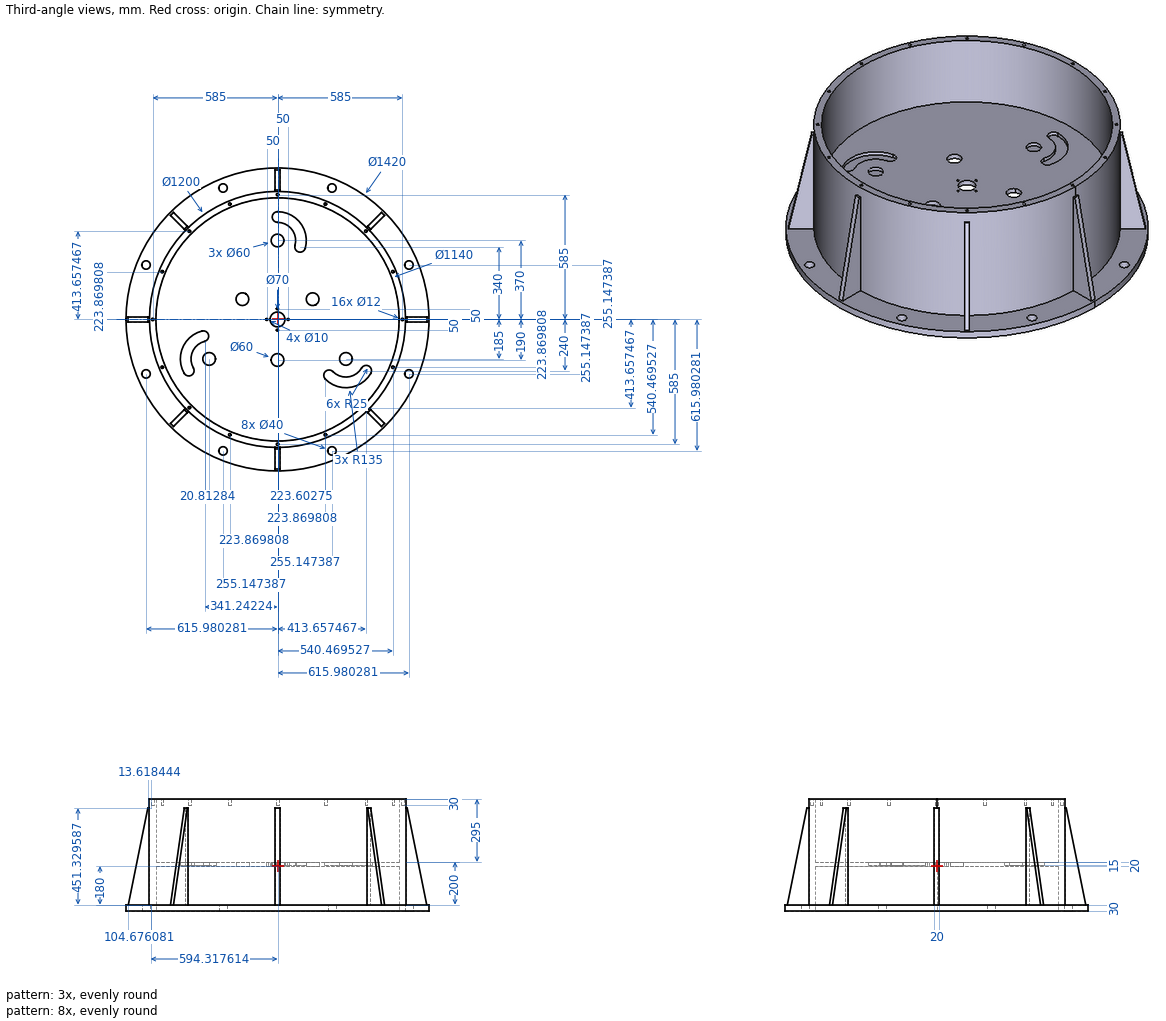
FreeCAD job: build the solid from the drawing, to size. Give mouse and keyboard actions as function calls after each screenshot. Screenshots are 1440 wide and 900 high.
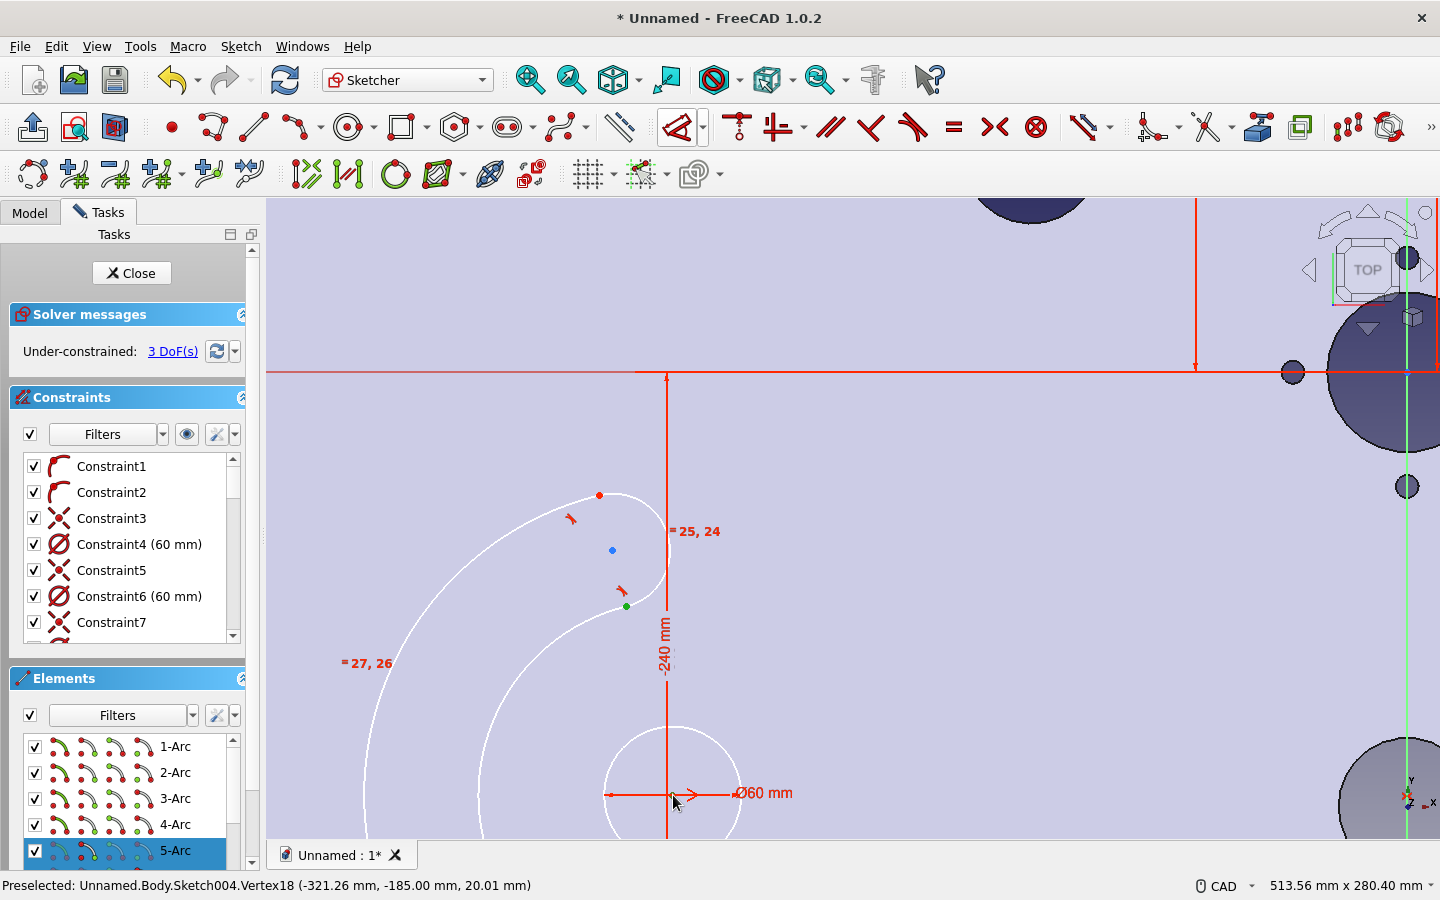
click(702, 128)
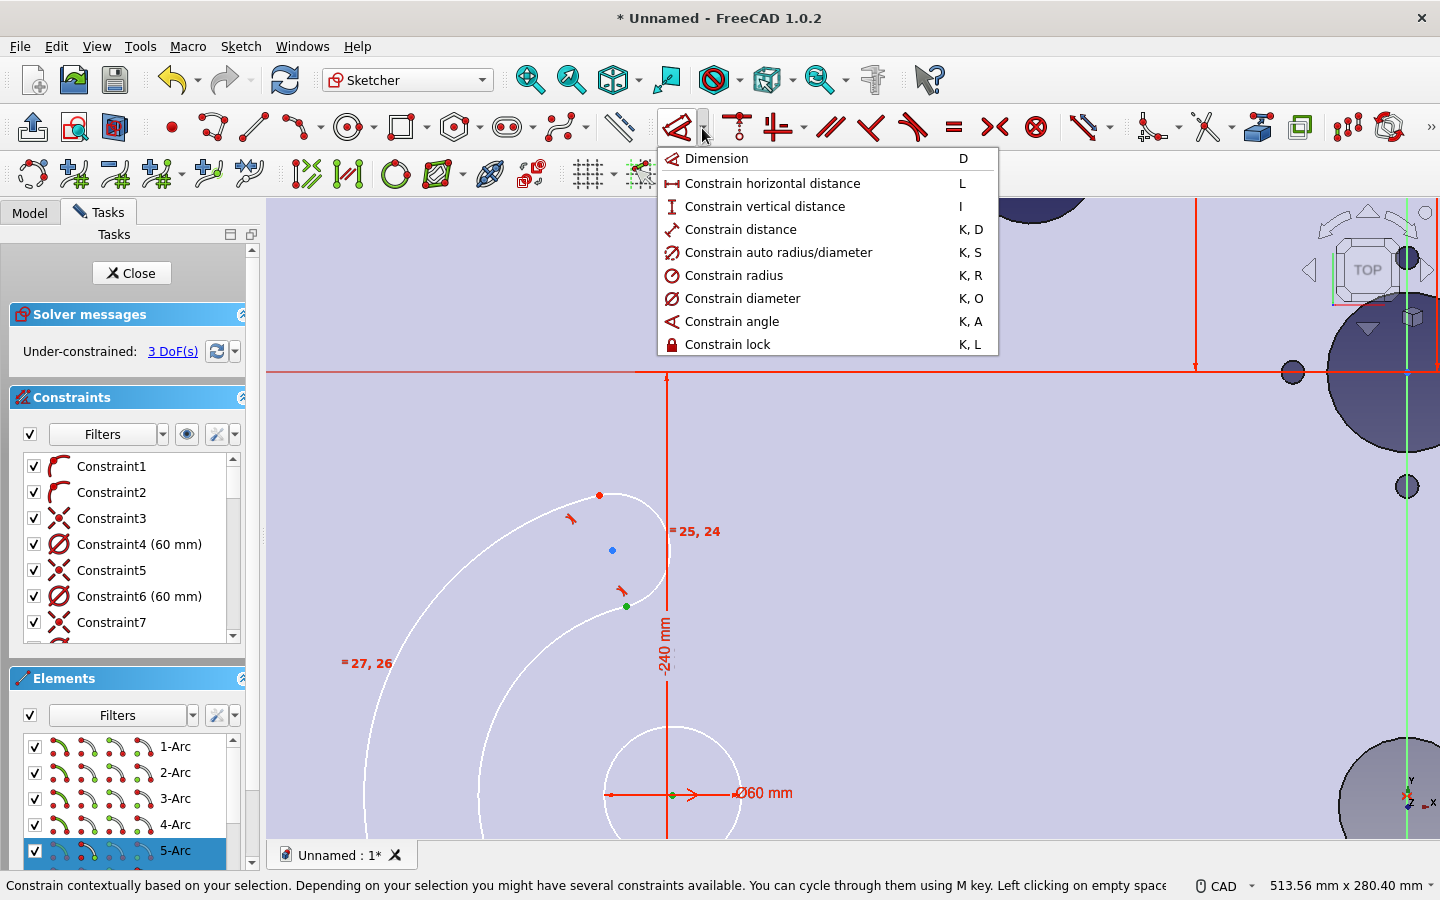
click(828, 184)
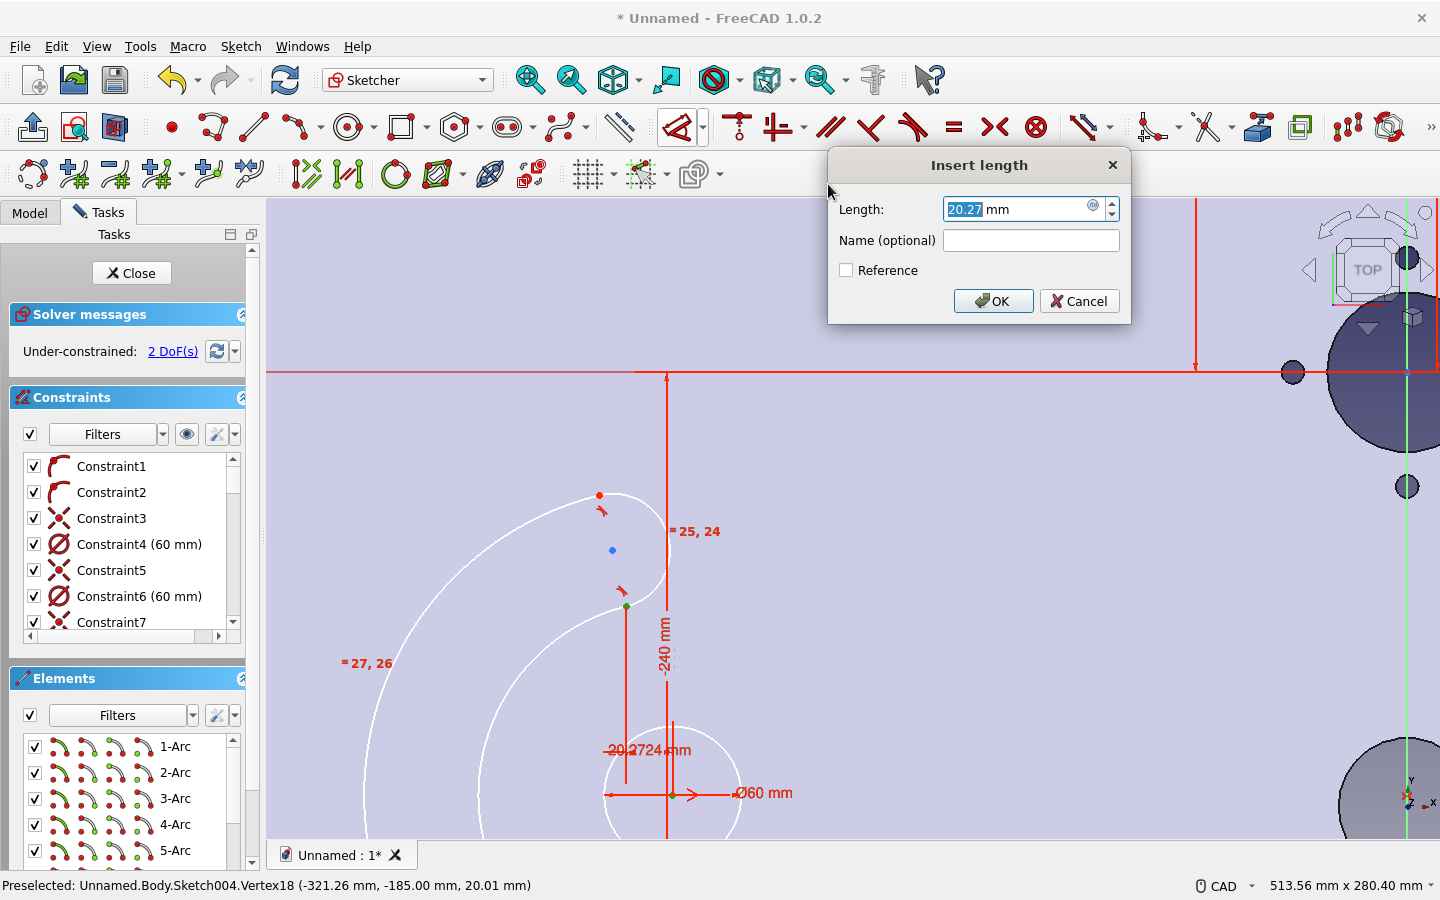
text(20.81284)
key(Return)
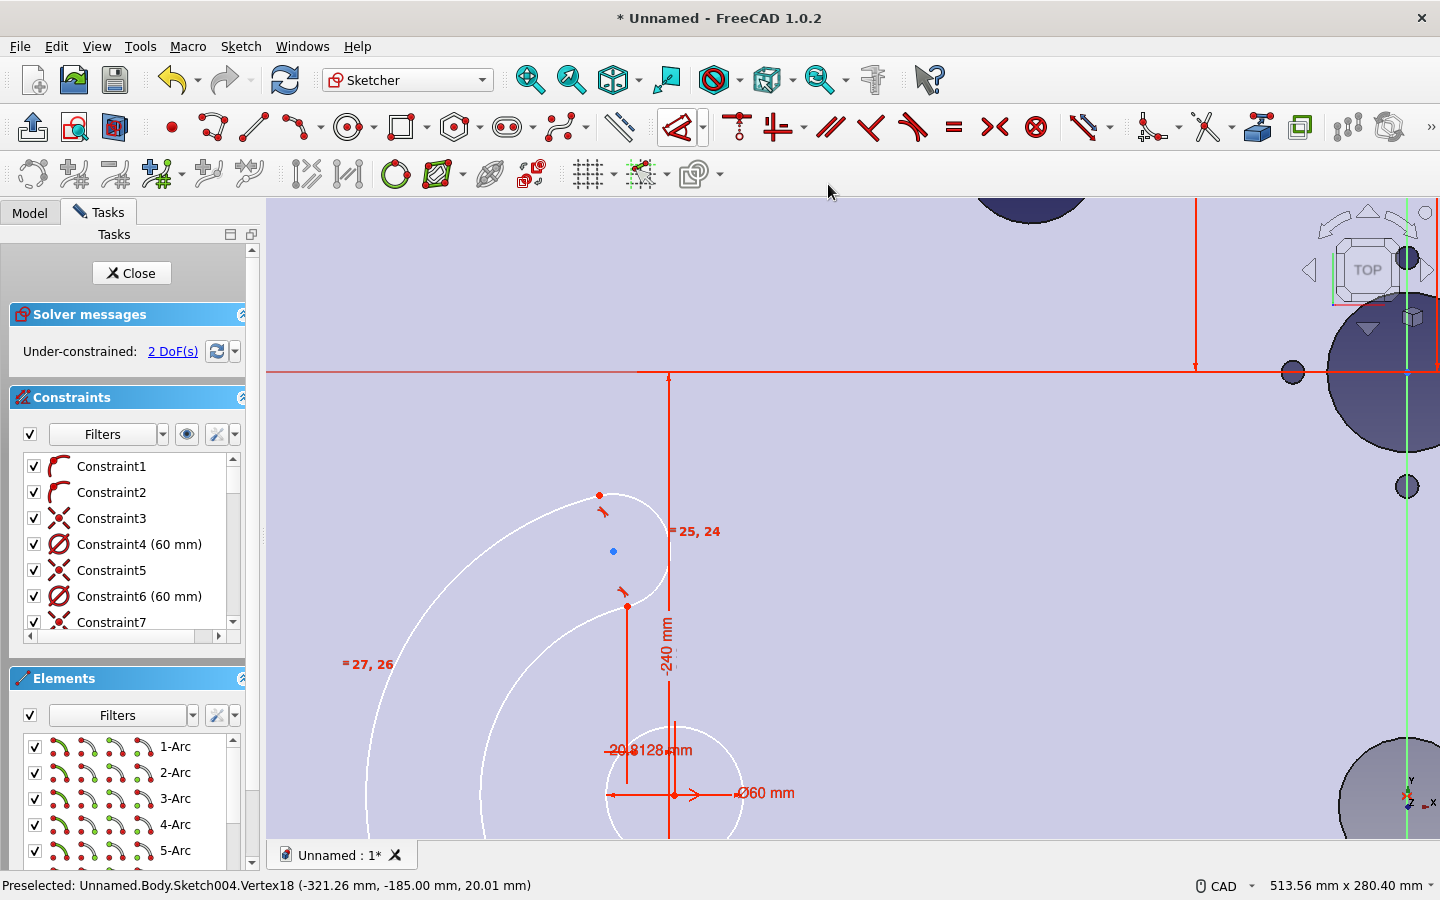
scroll(629, 609, down, 8)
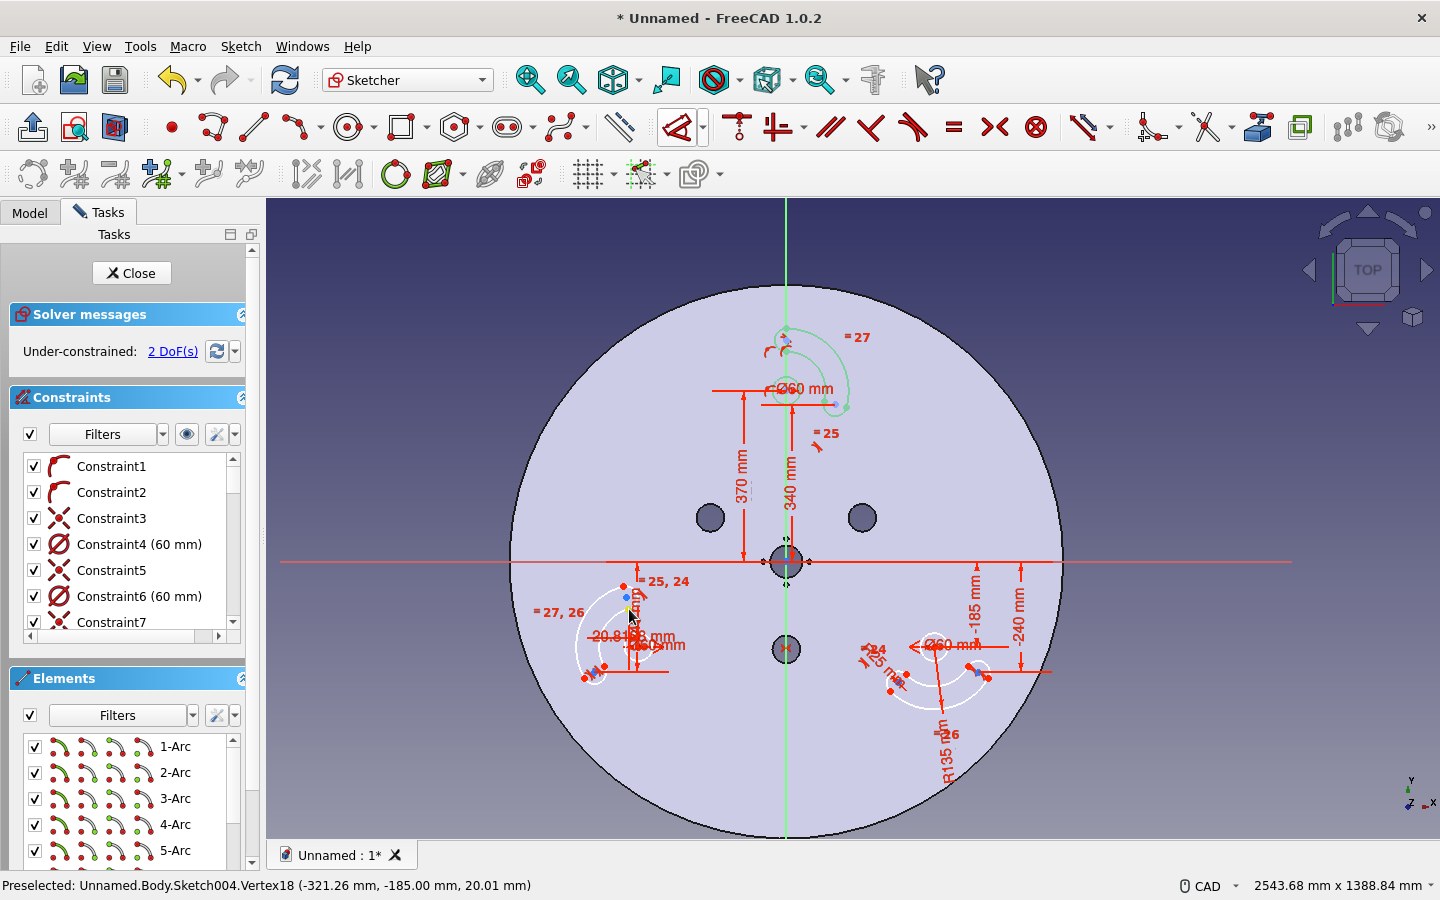
click(890, 691)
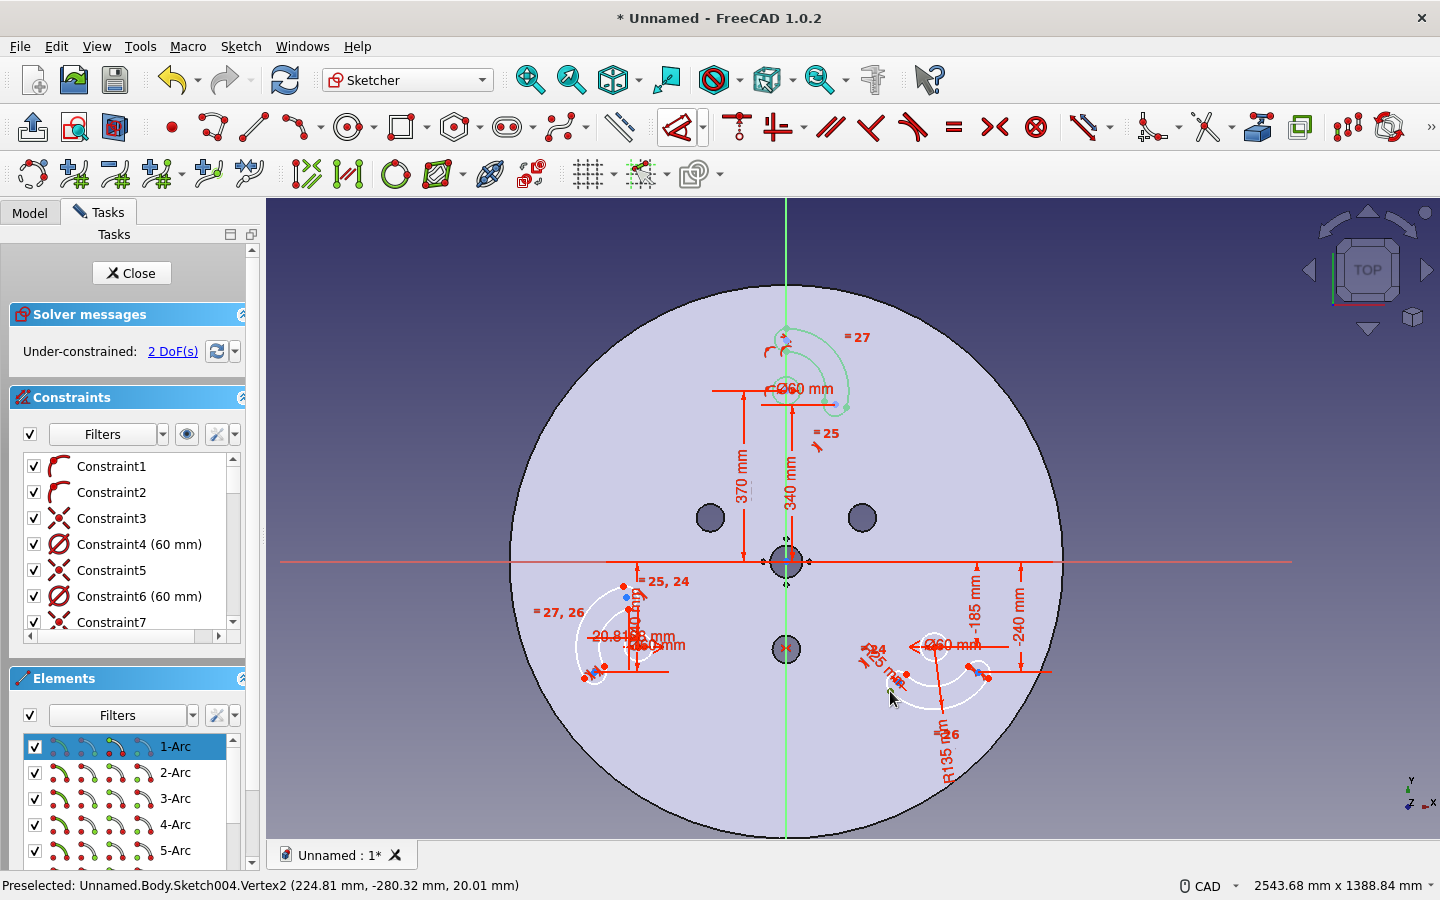
key(l)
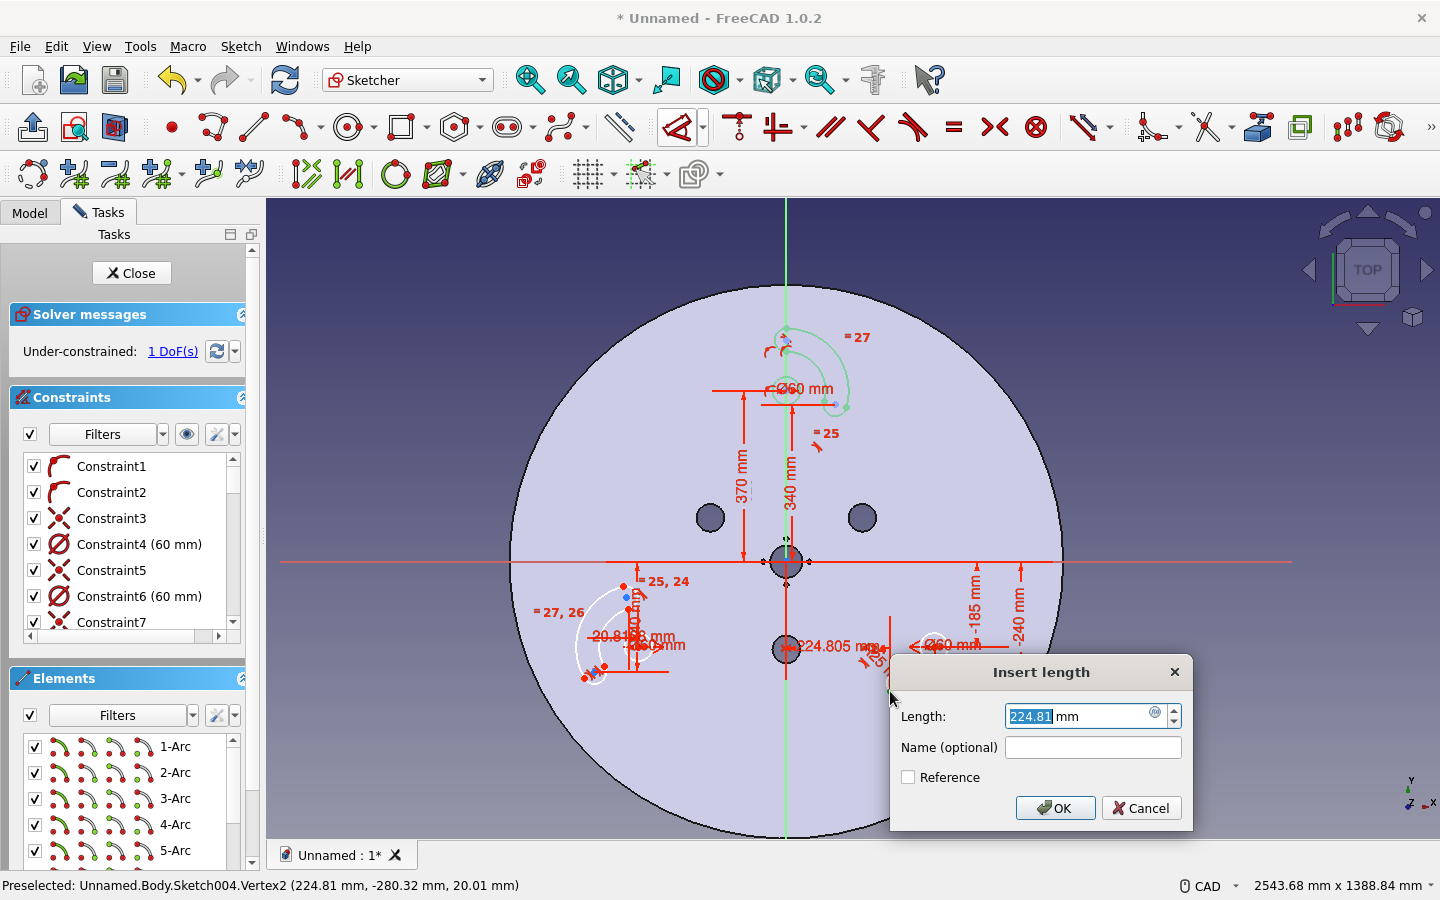
text(223.60275)
key(Return)